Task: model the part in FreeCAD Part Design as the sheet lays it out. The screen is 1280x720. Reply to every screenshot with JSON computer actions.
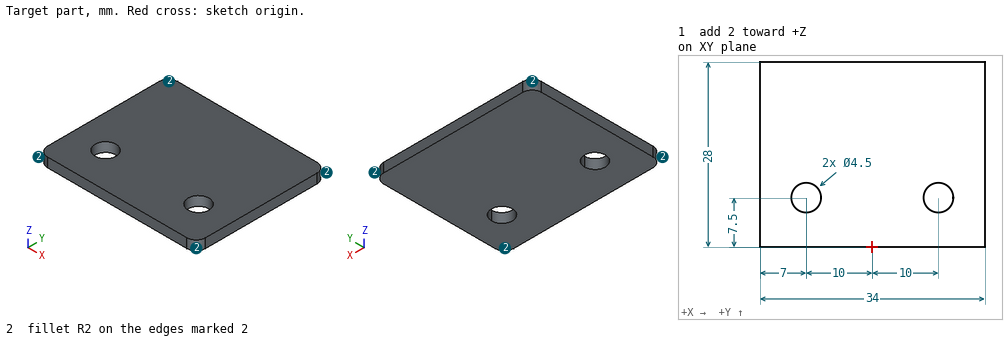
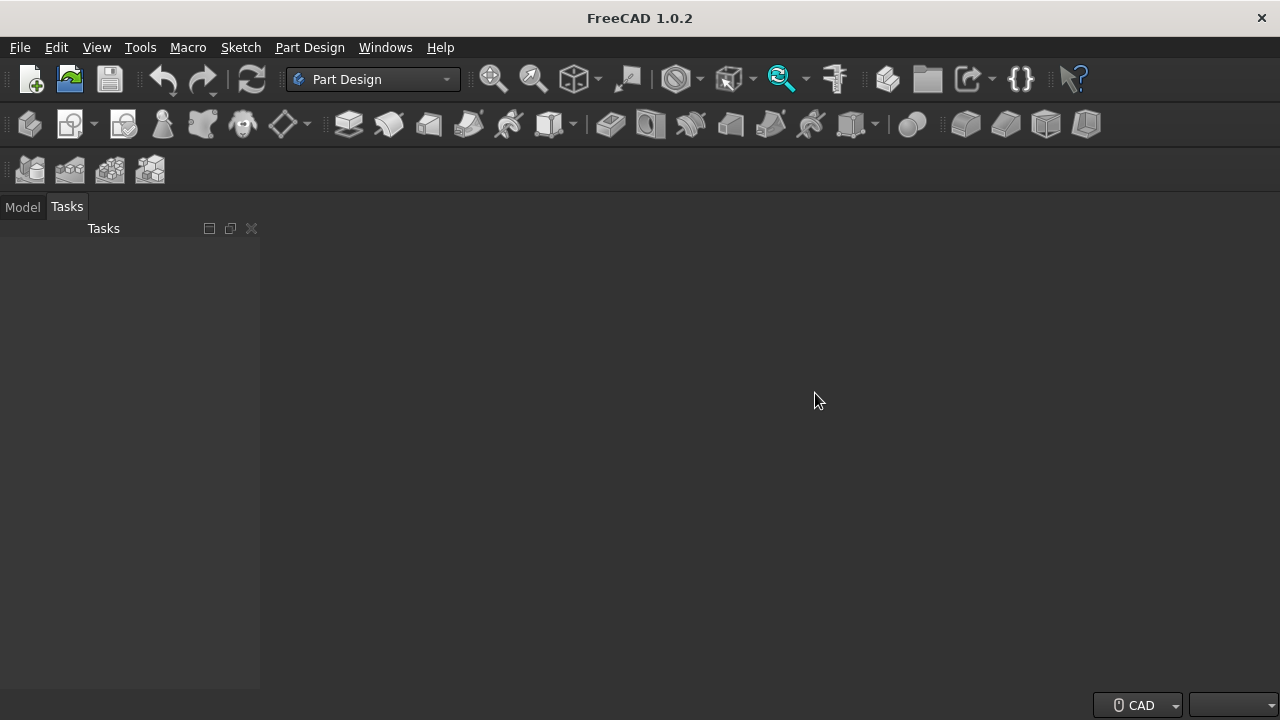
{"action": "key", "text": "ctrl+n"}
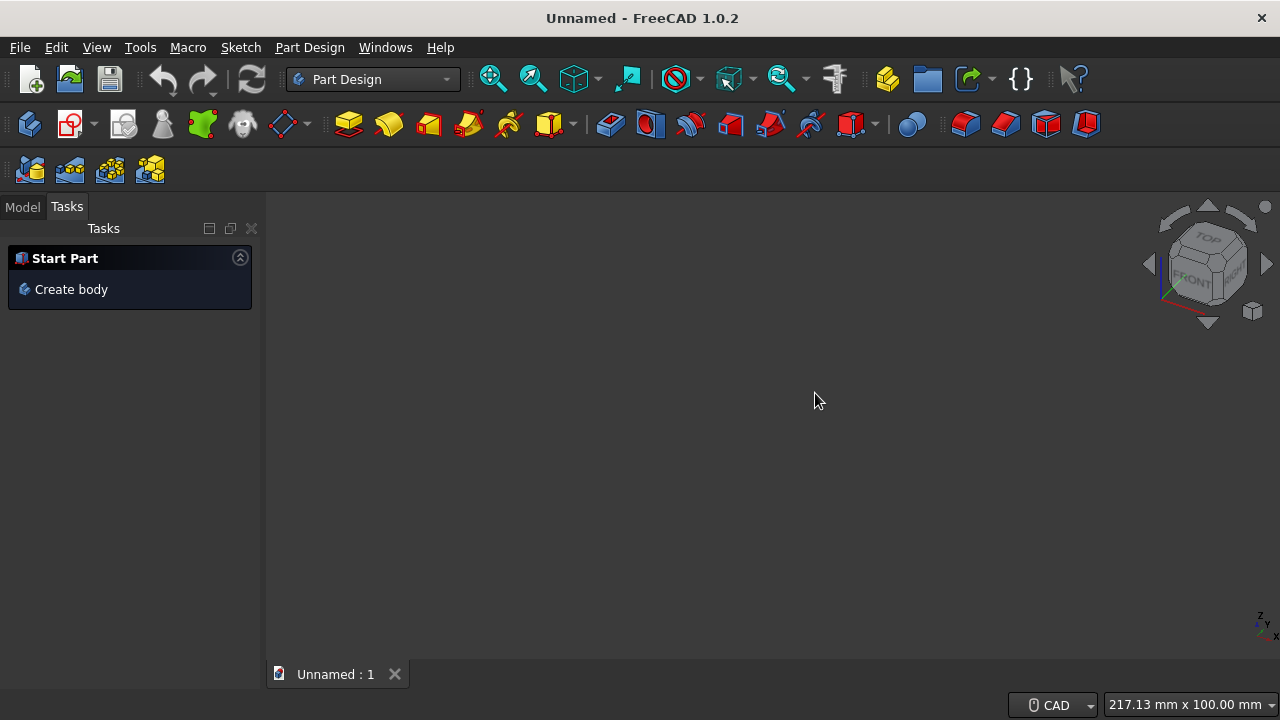
{"action": "left_click", "coordinate": [70, 124]}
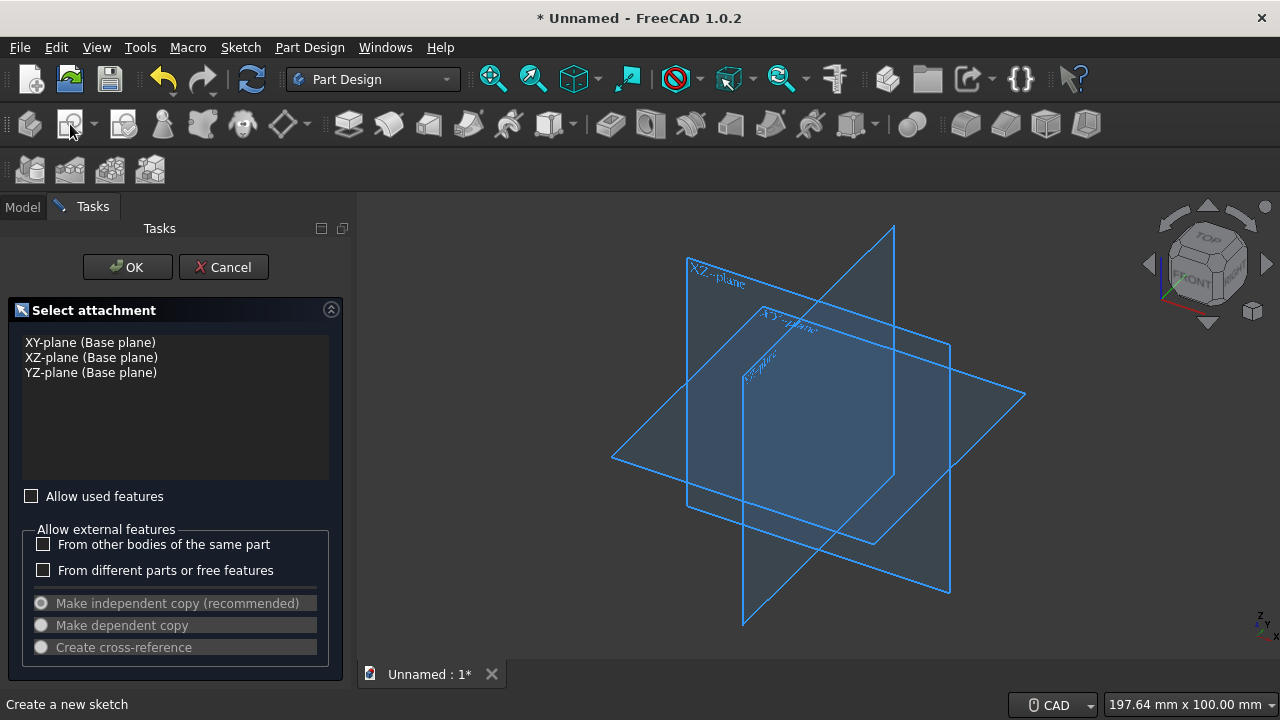
{"action": "left_click", "coordinate": [82, 342]}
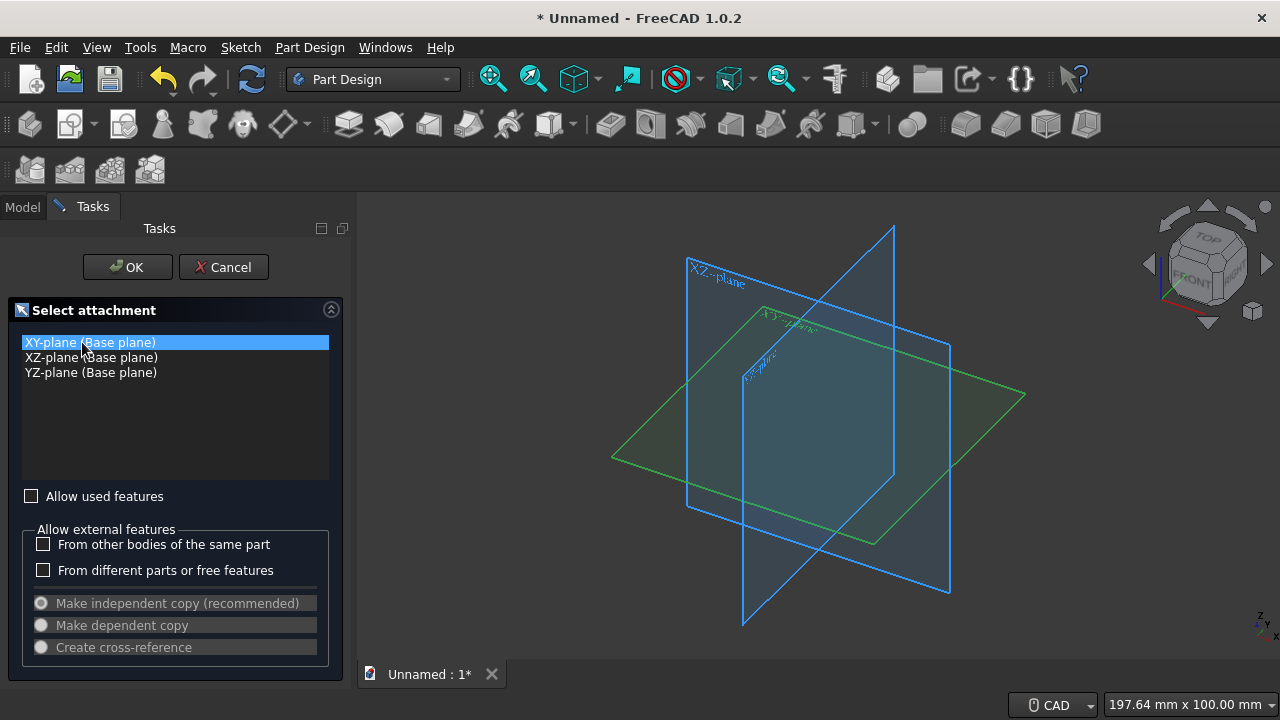
{"action": "left_click", "coordinate": [128, 267]}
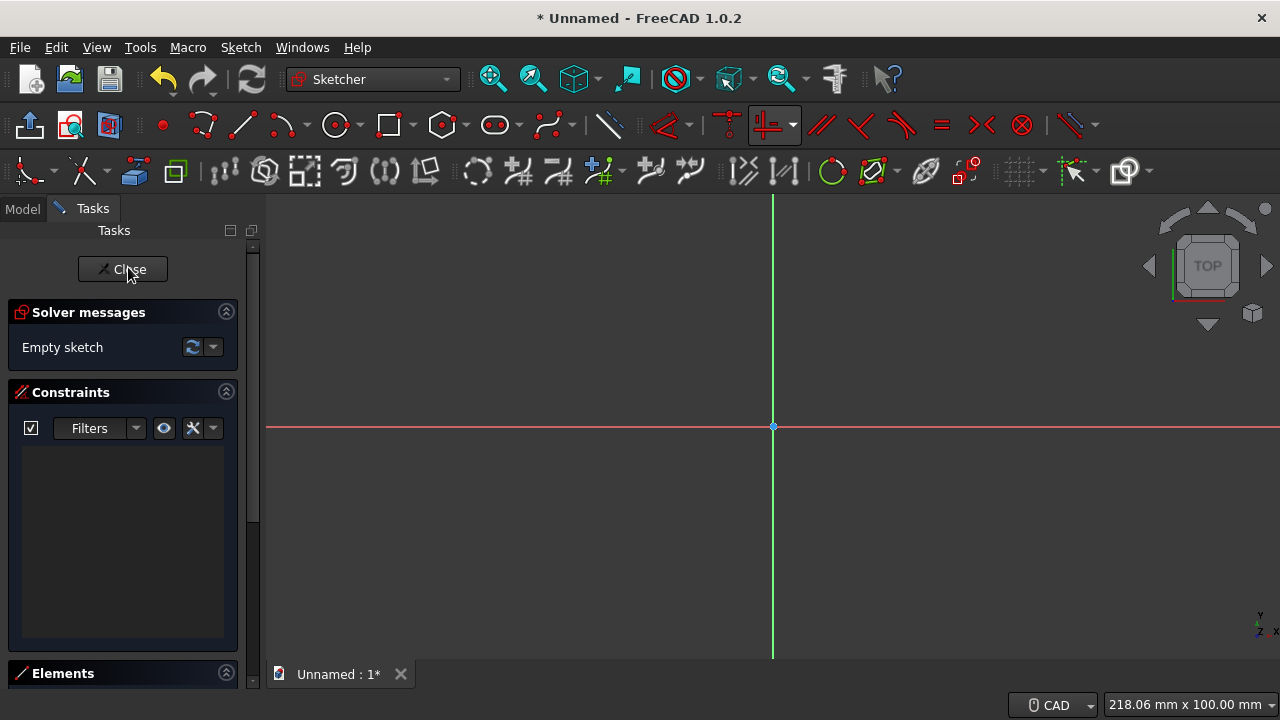
{"action": "scroll", "coordinate": [829, 308], "scroll_direction": "up", "scroll_amount": 4}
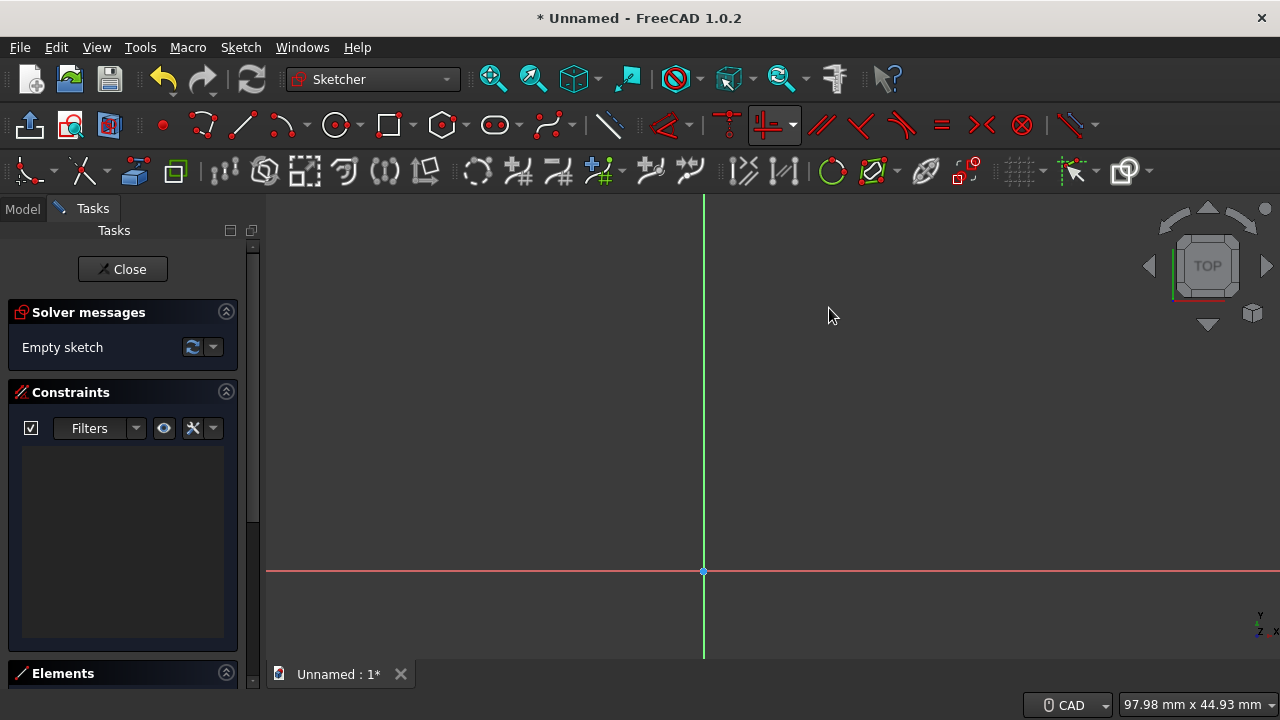
{"action": "key", "text": "g r"}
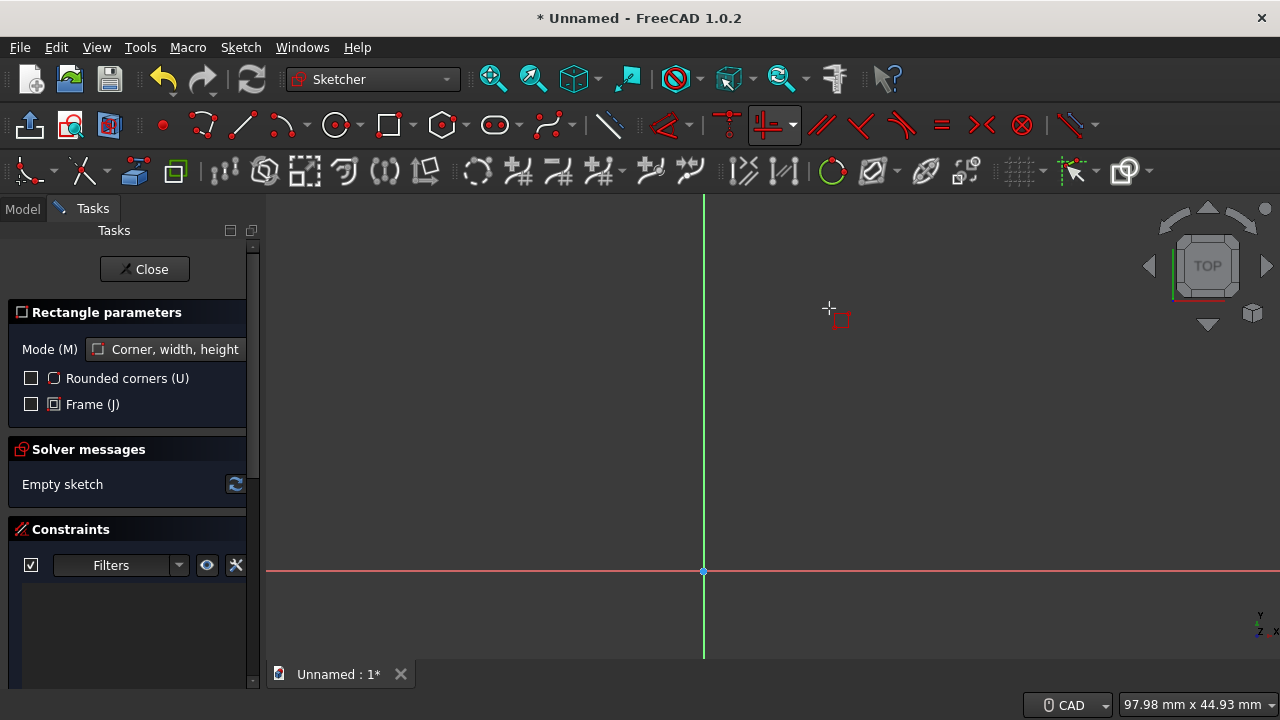
{"action": "left_click", "coordinate": [528, 282]}
{"action": "left_click", "coordinate": [880, 571]}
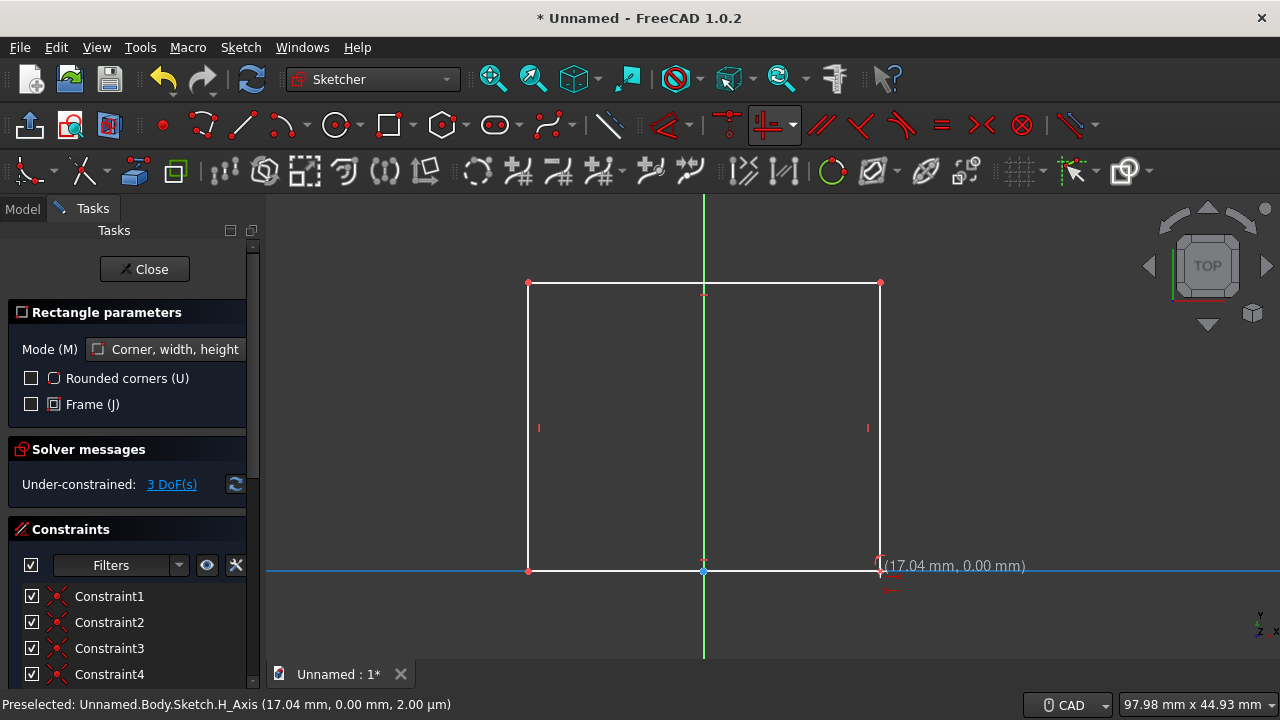
{"action": "left_click", "coordinate": [336, 126]}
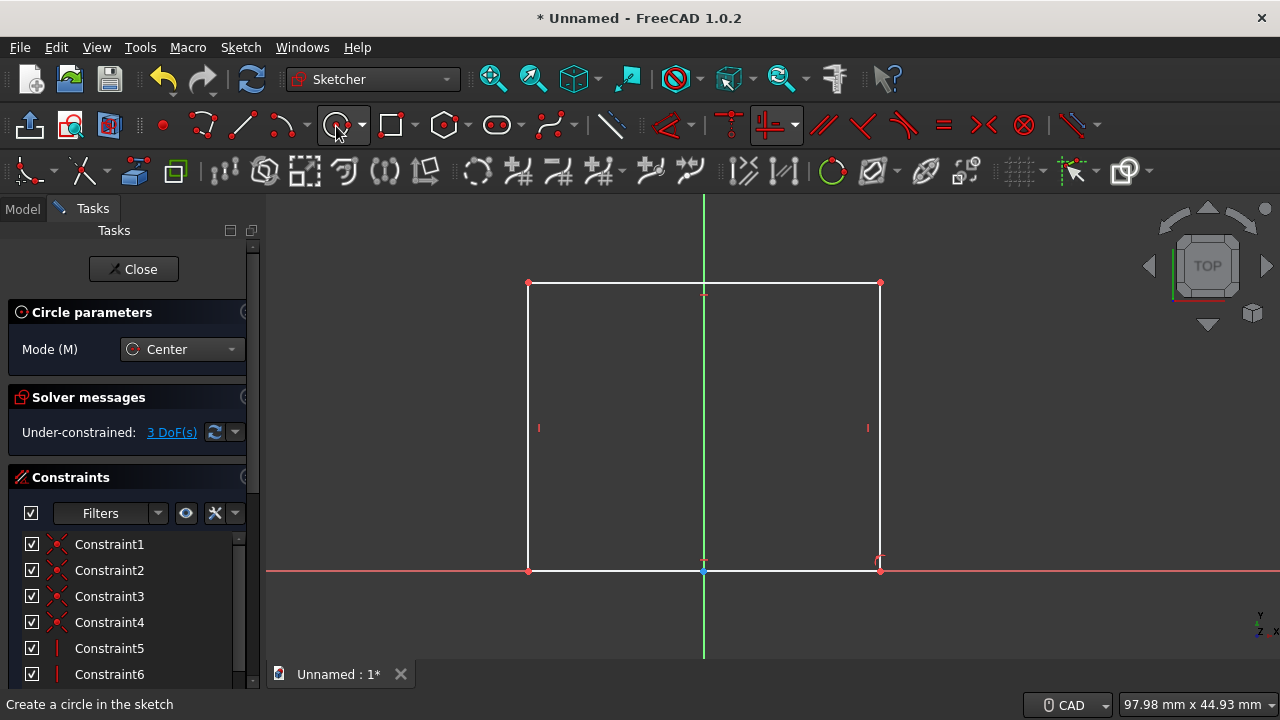
{"action": "left_click", "coordinate": [600, 494]}
{"action": "mouse_move", "coordinate": [617, 477]}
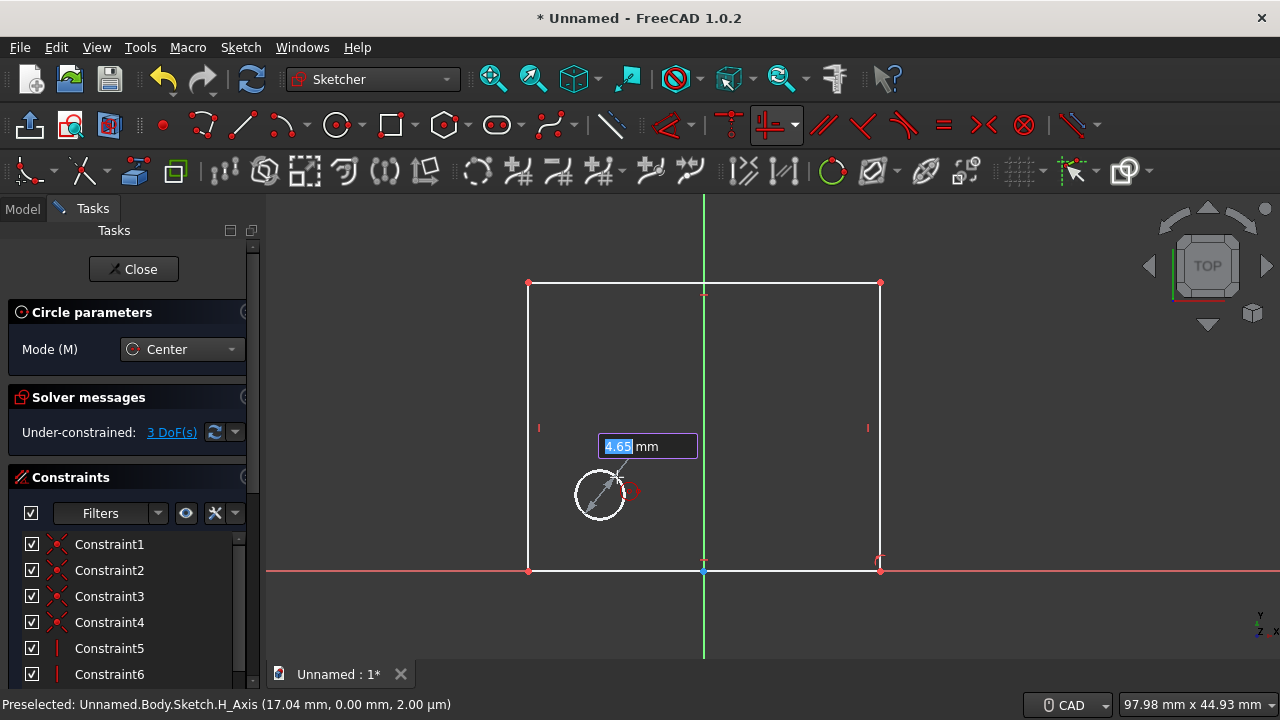
{"action": "type", "text": "4.5"}
{"action": "key", "text": "Return"}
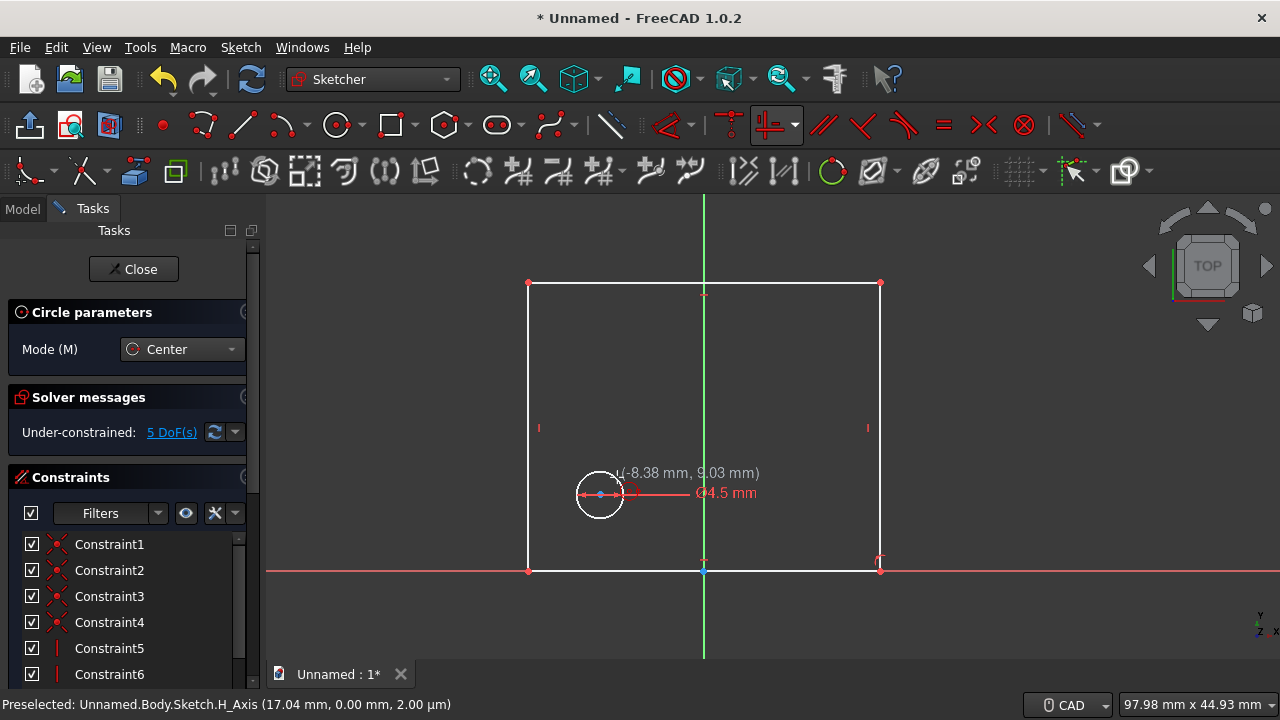
{"action": "left_click", "coordinate": [807, 494]}
{"action": "mouse_move", "coordinate": [824, 477]}